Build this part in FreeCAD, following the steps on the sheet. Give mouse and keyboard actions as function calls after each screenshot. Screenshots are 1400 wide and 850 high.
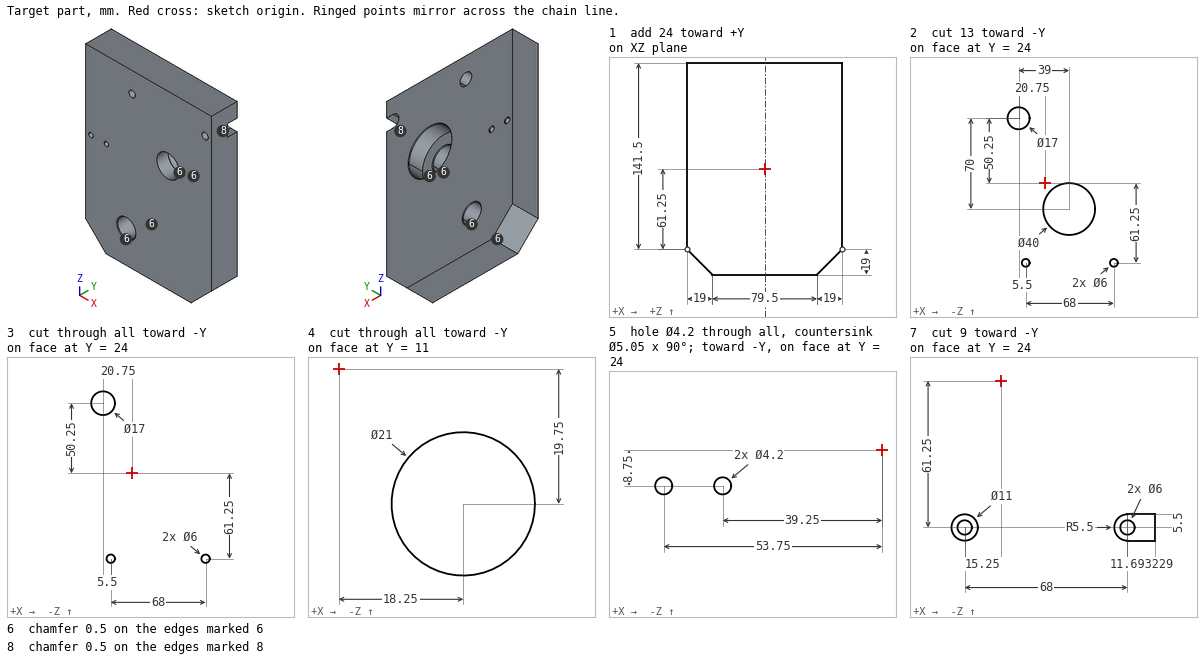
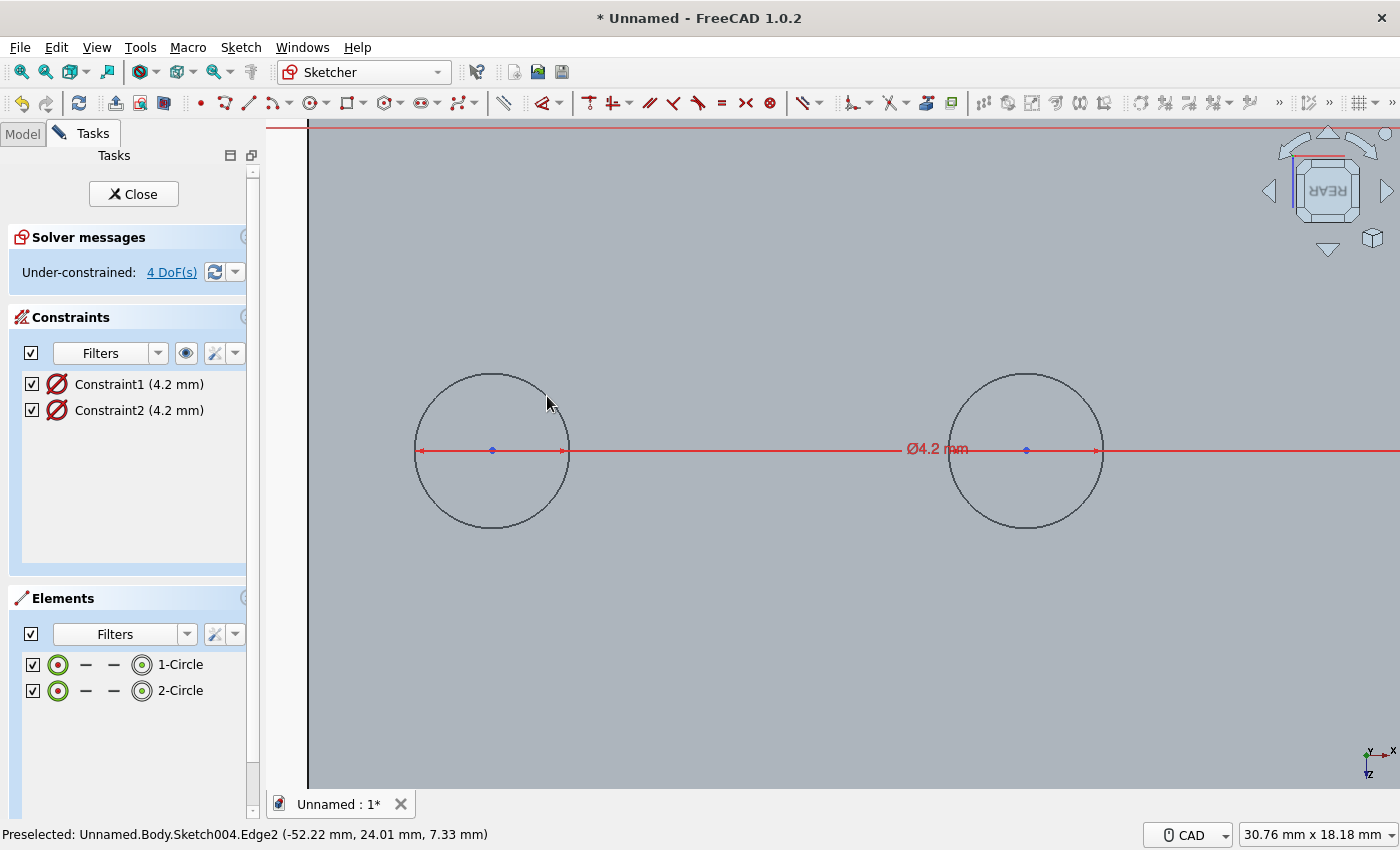
click(1026, 451)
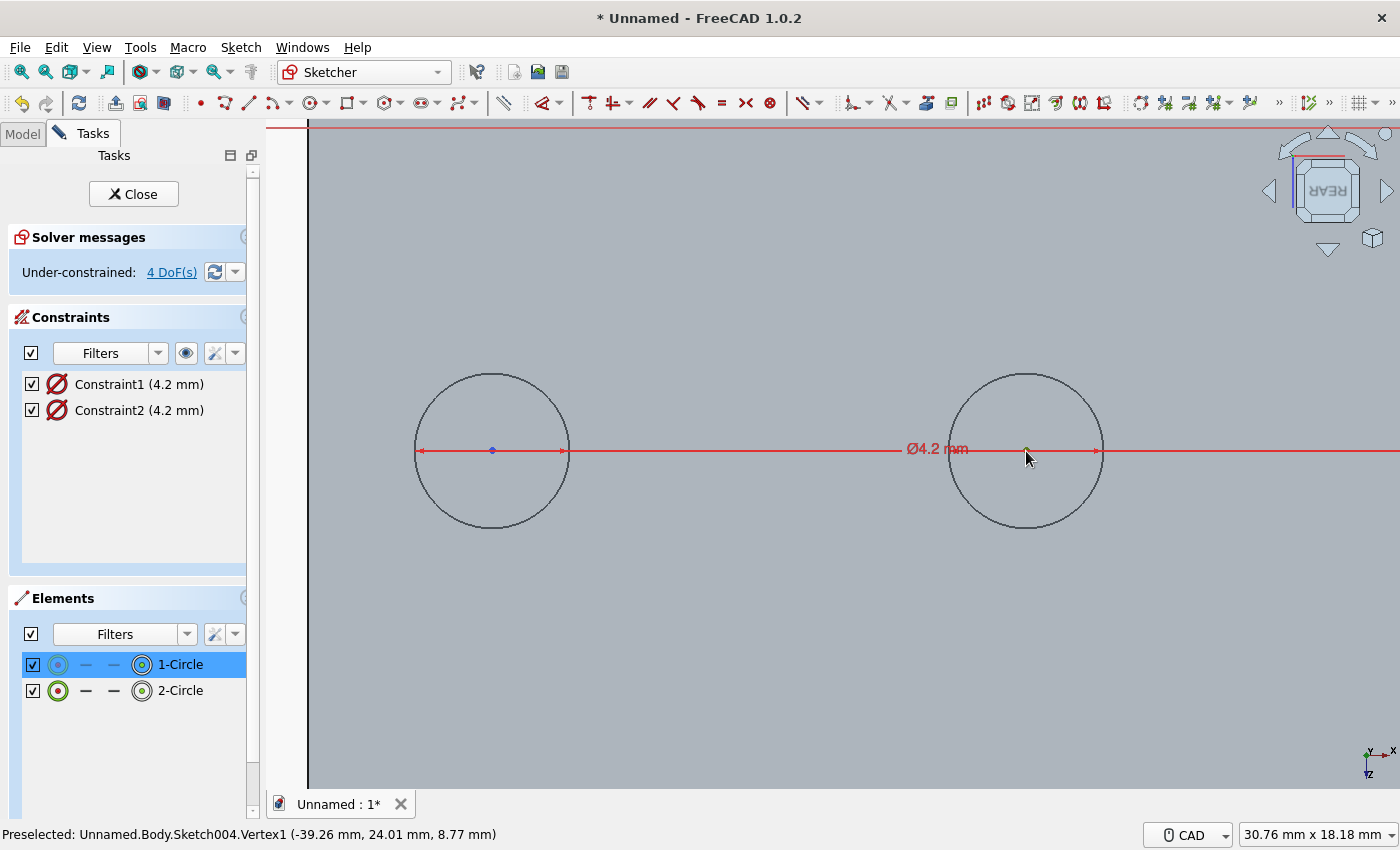
click(492, 451)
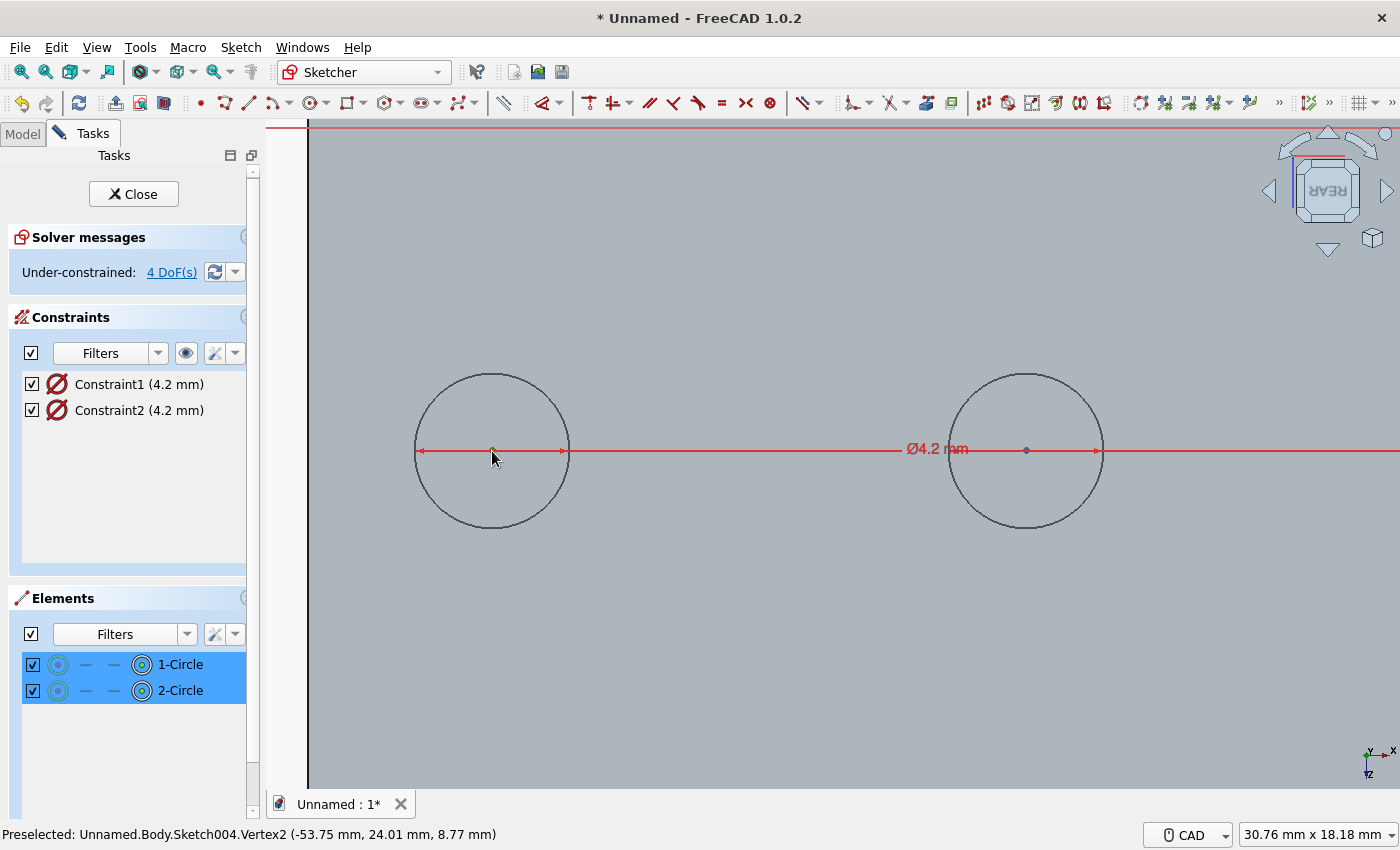
key(h)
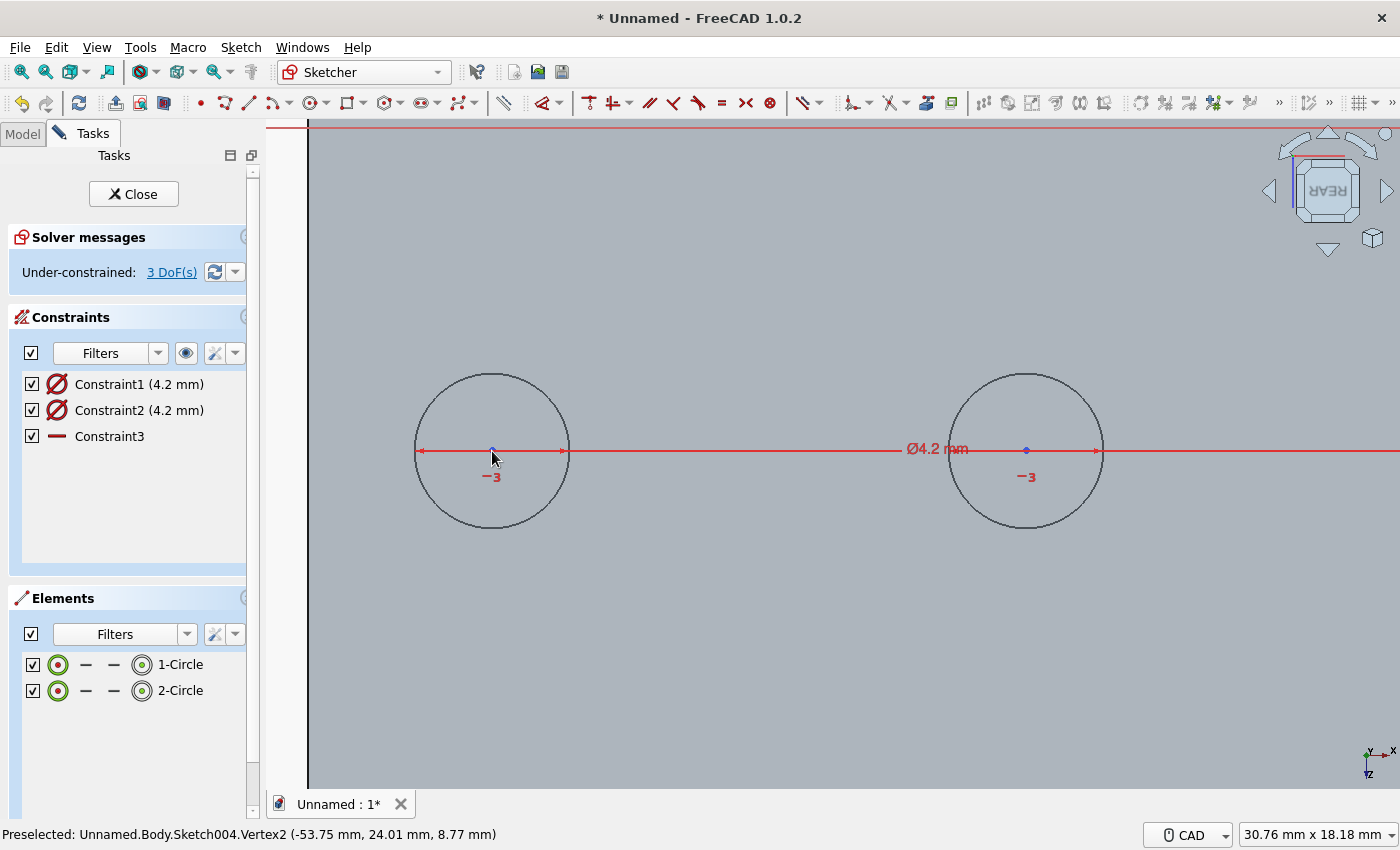
key(d)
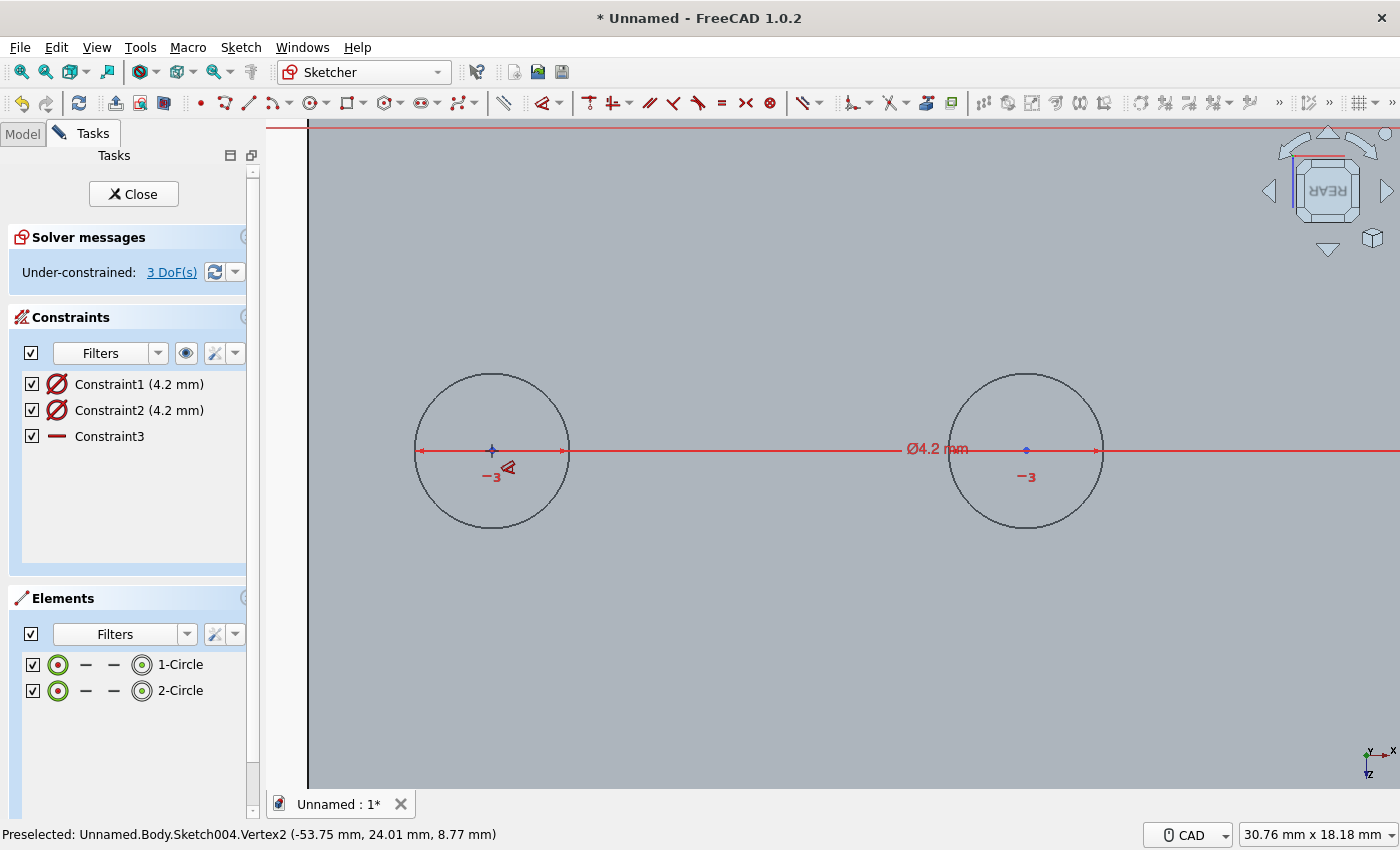
click(1026, 451)
click(992, 299)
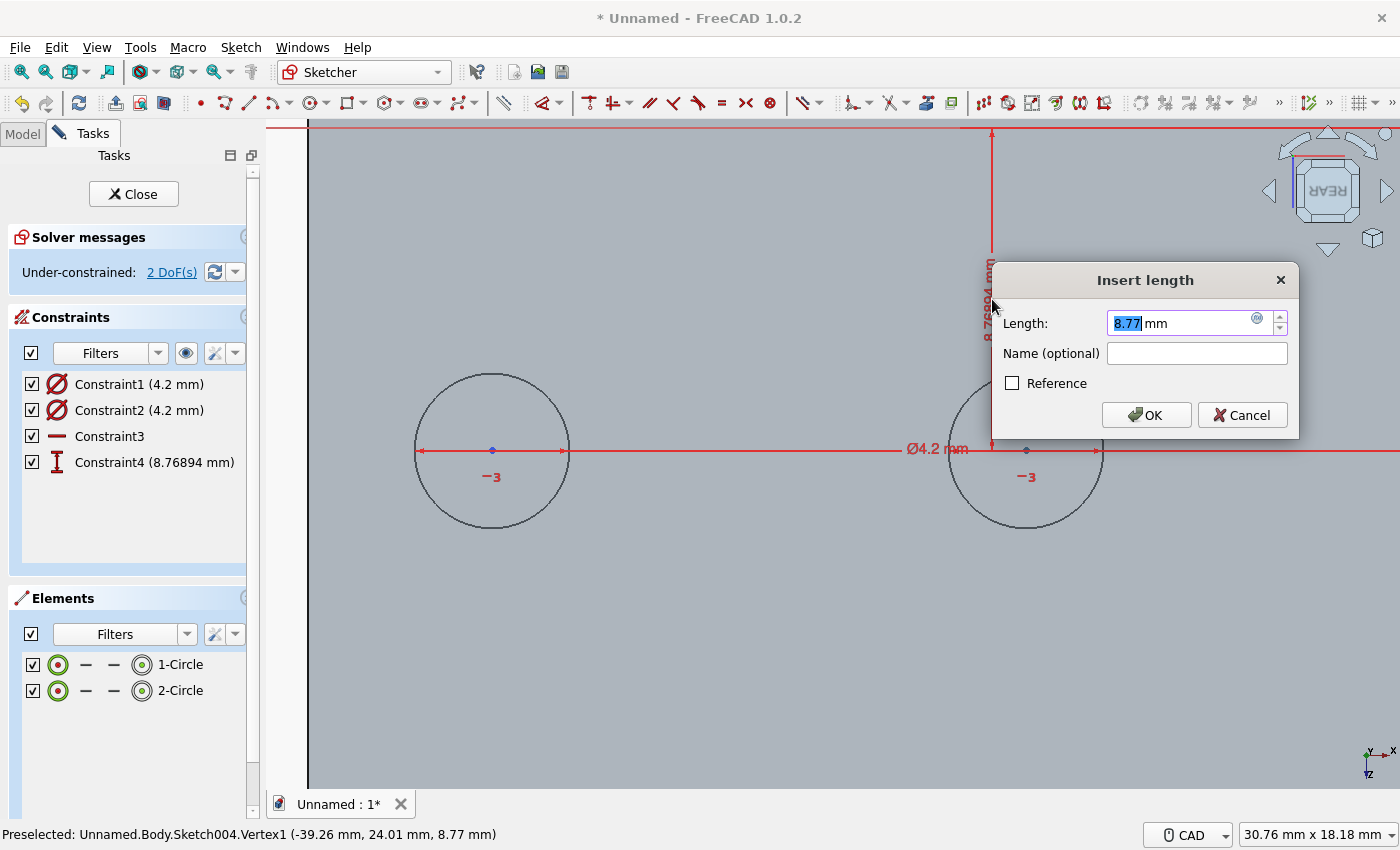
text(8.75)
key(Return)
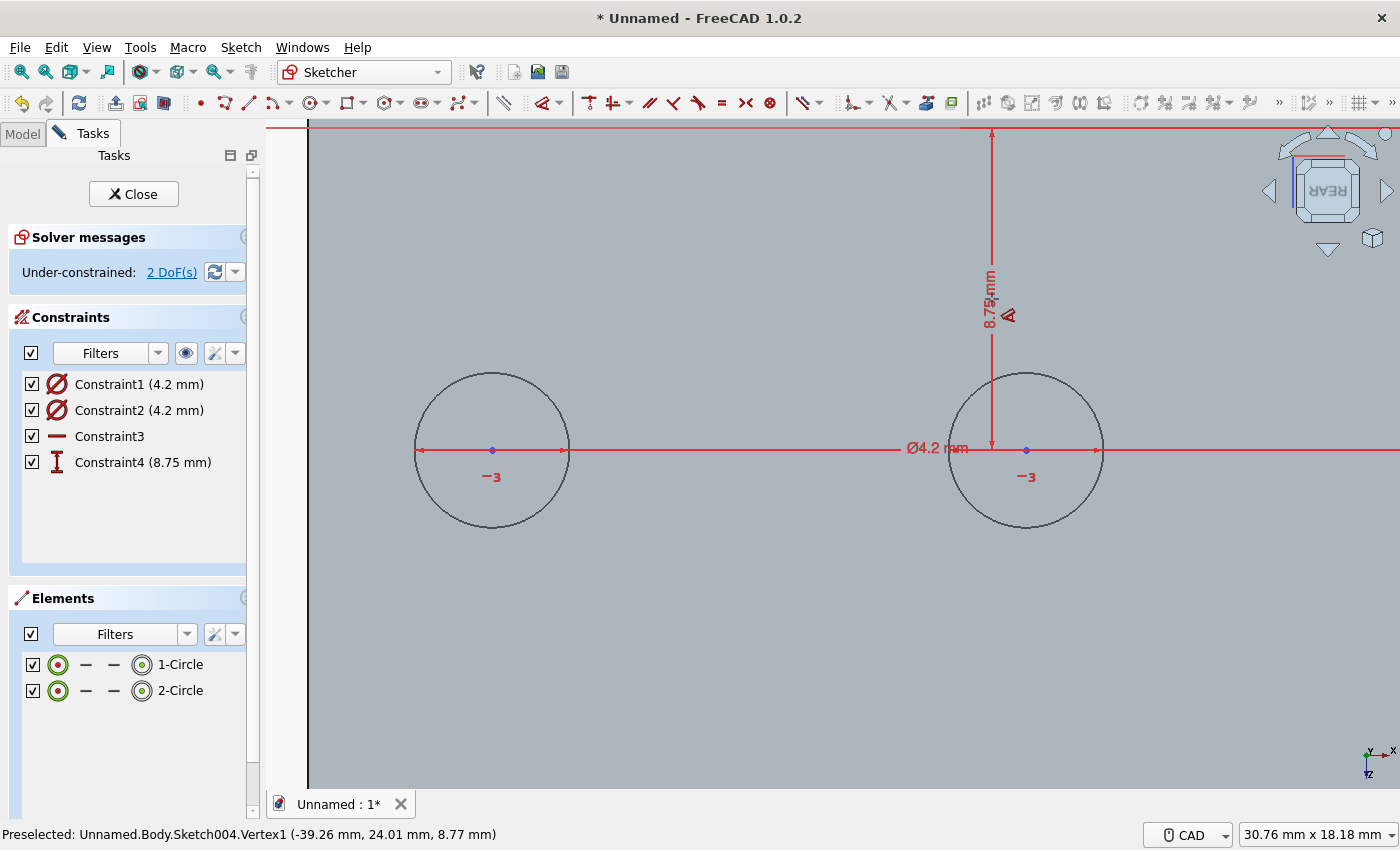
click(1026, 450)
click(1131, 484)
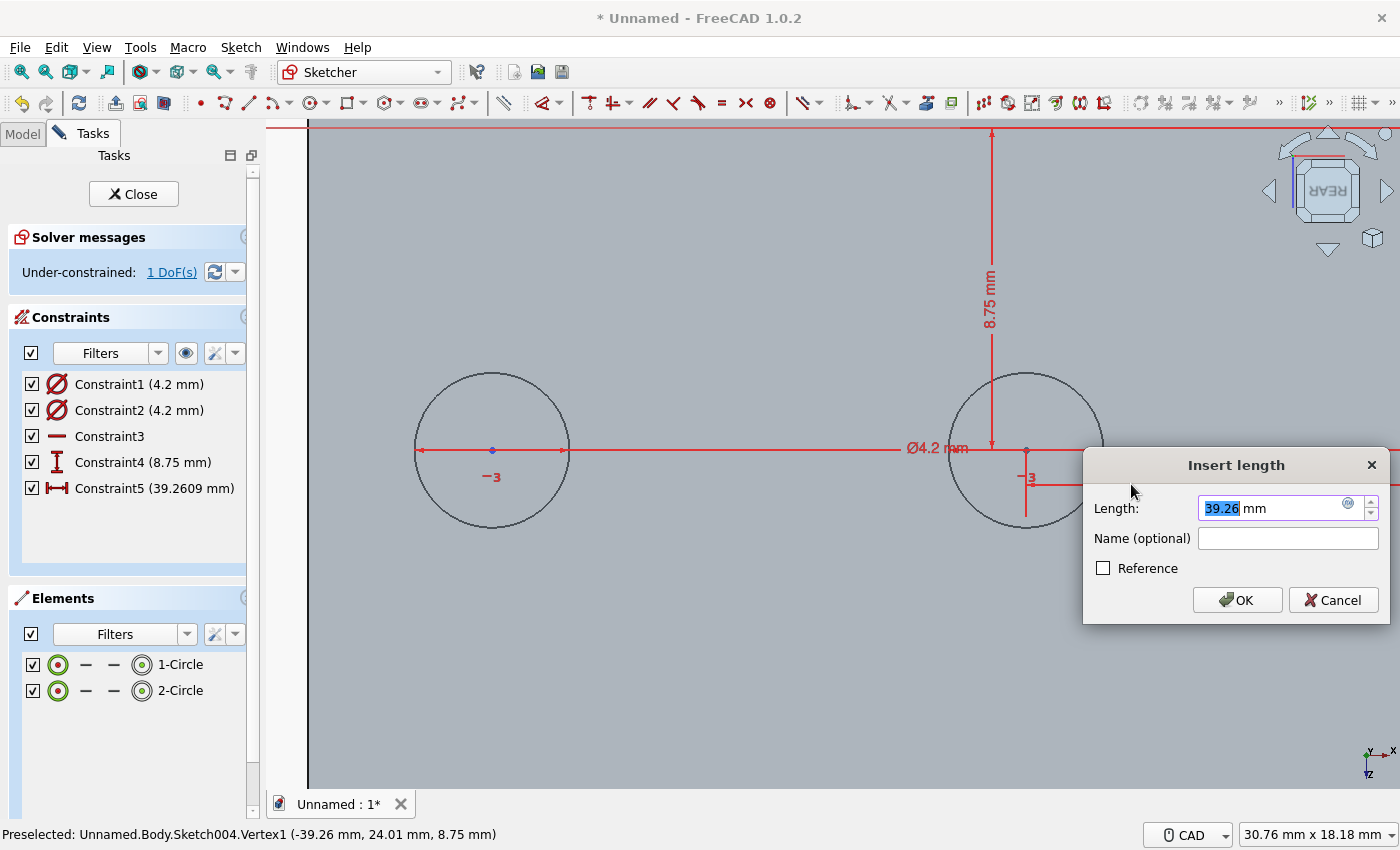
text(39.25)
key(Return)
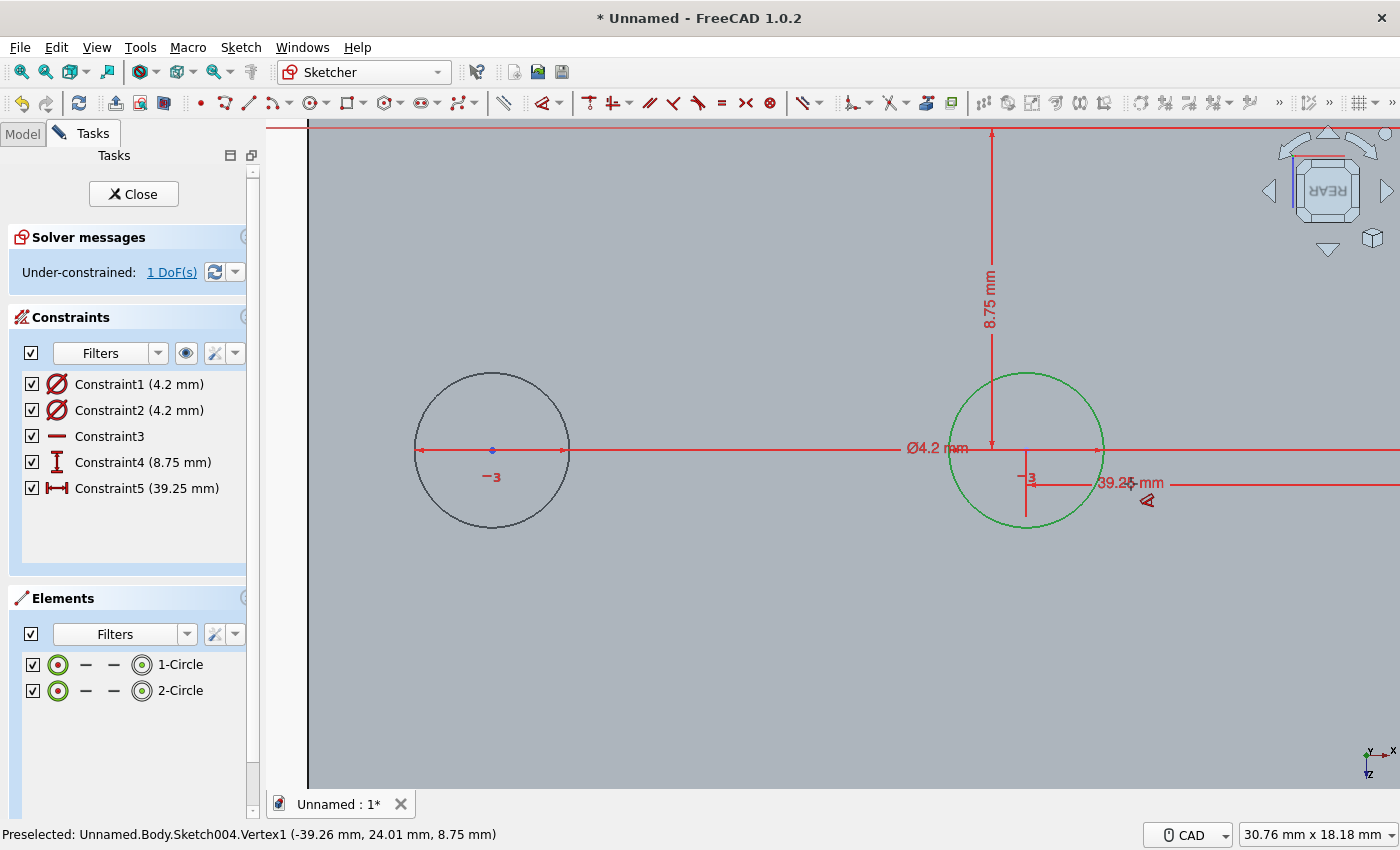
click(492, 450)
click(863, 484)